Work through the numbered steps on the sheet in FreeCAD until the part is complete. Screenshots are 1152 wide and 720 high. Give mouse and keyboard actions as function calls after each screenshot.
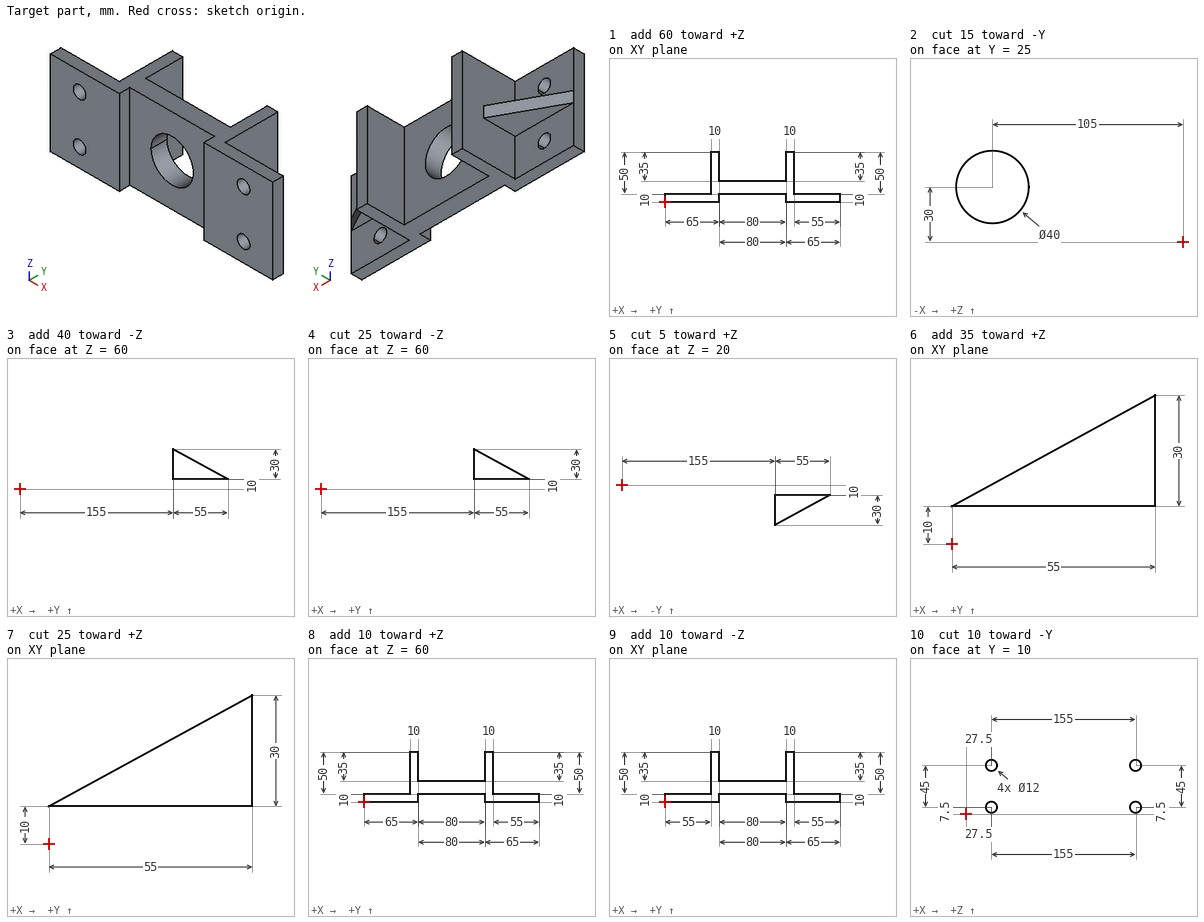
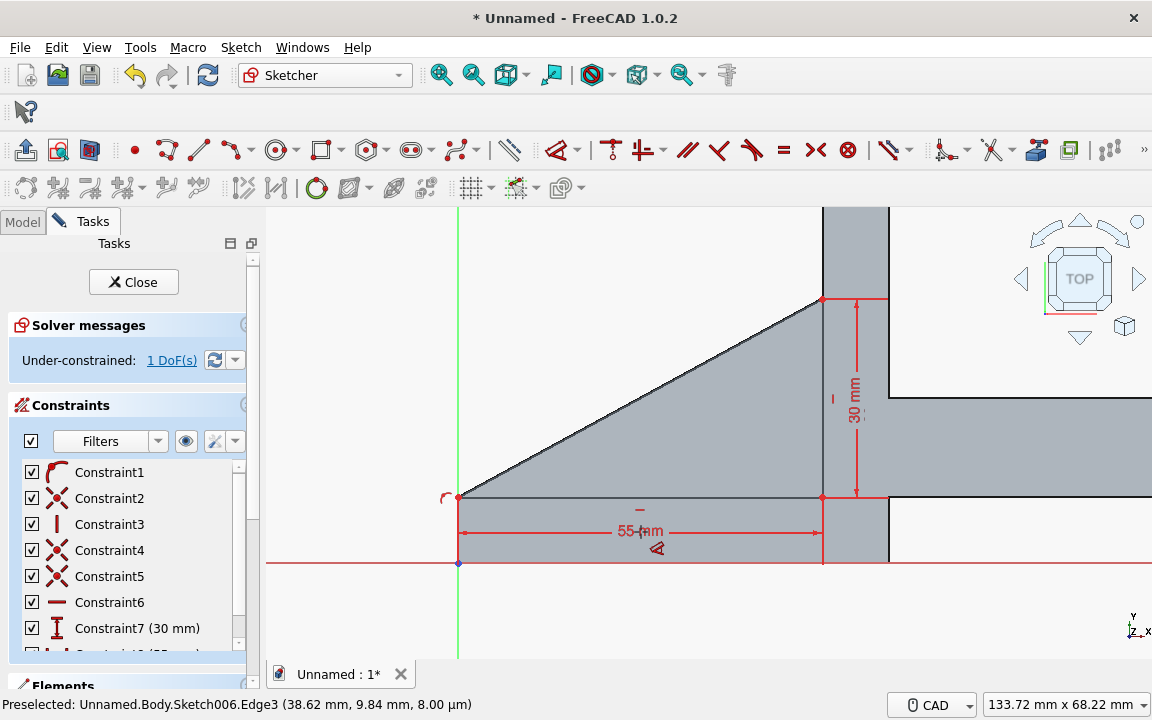
click(458, 498)
click(424, 531)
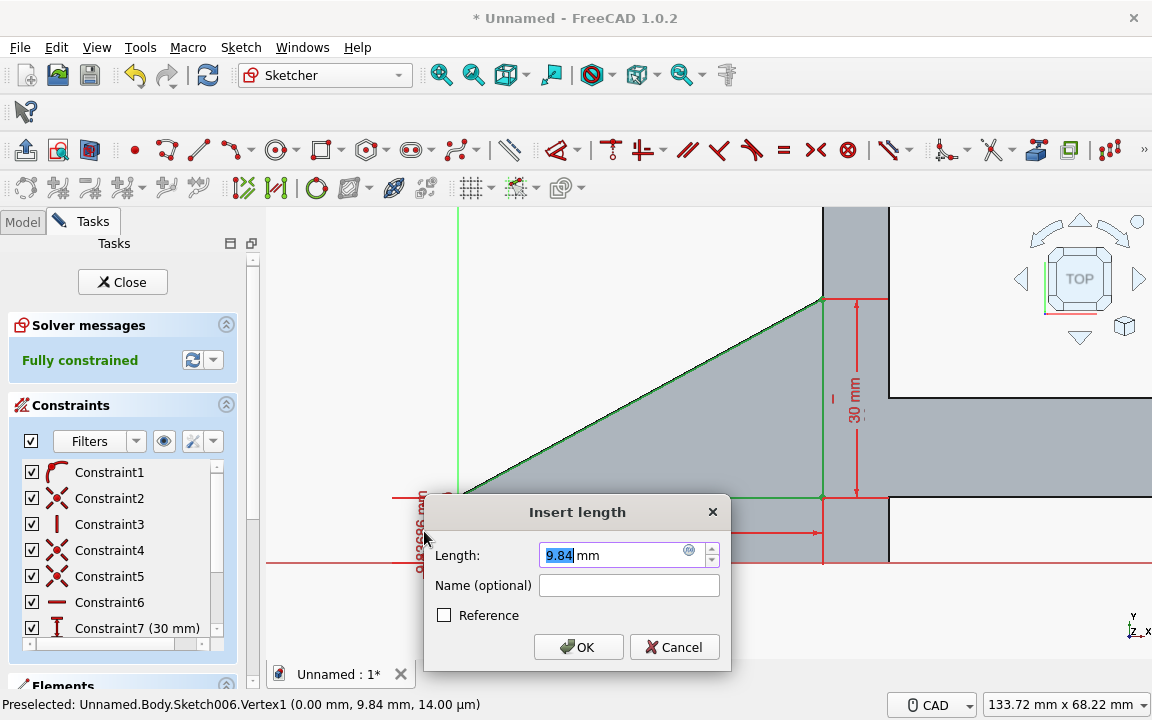
text(10)
key(Return)
key(Escape)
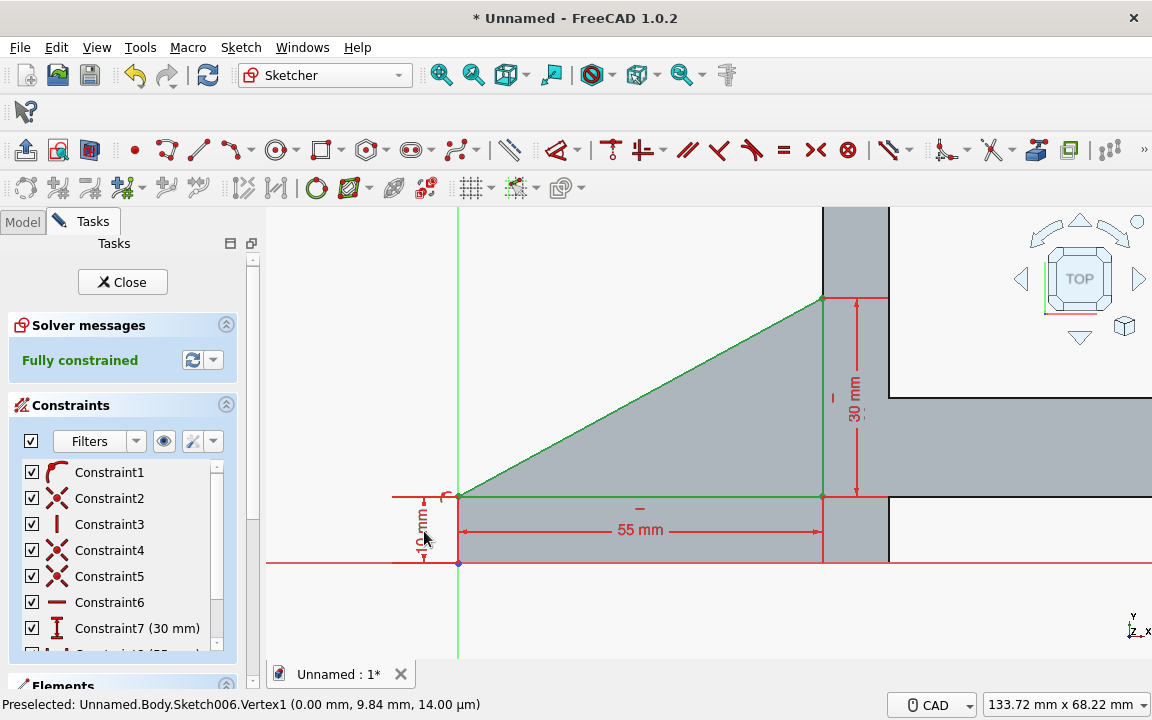
click(123, 282)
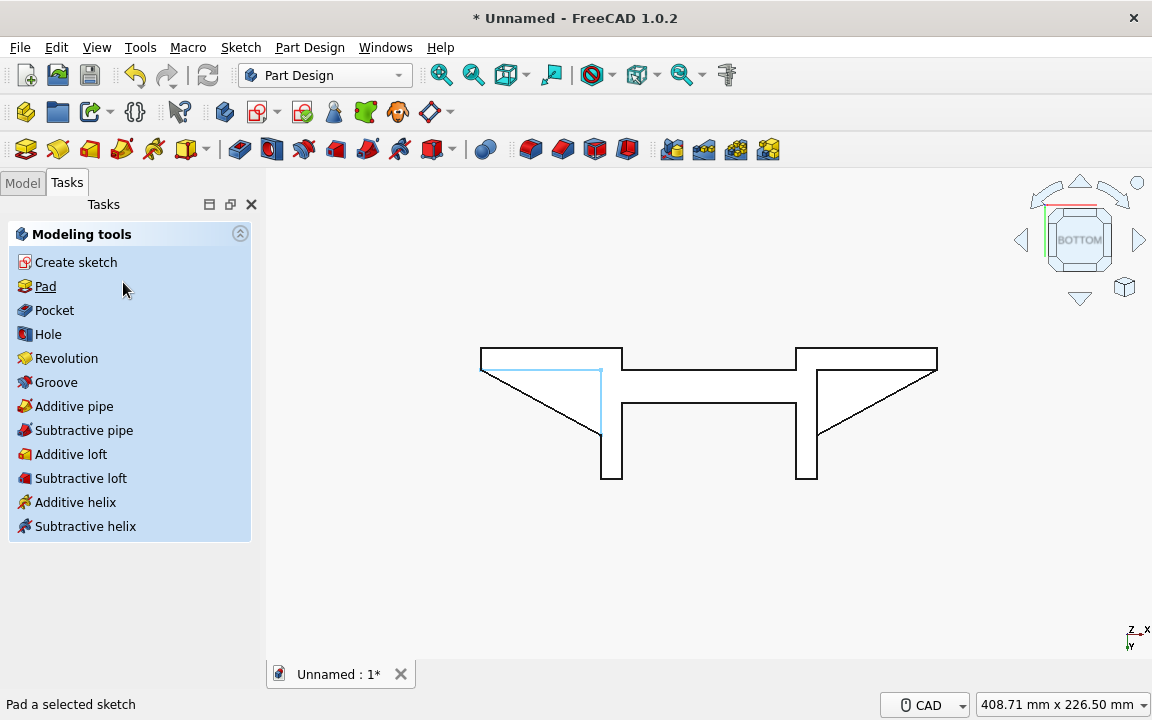
click(240, 150)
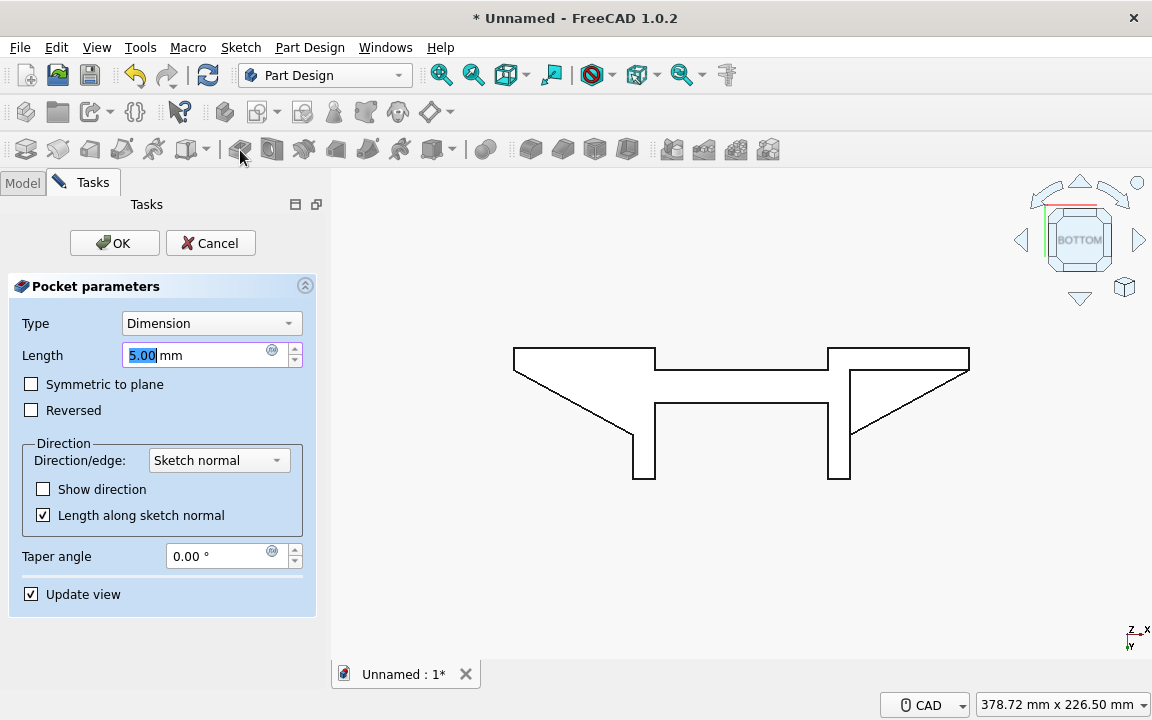
text(25)
key(Tab)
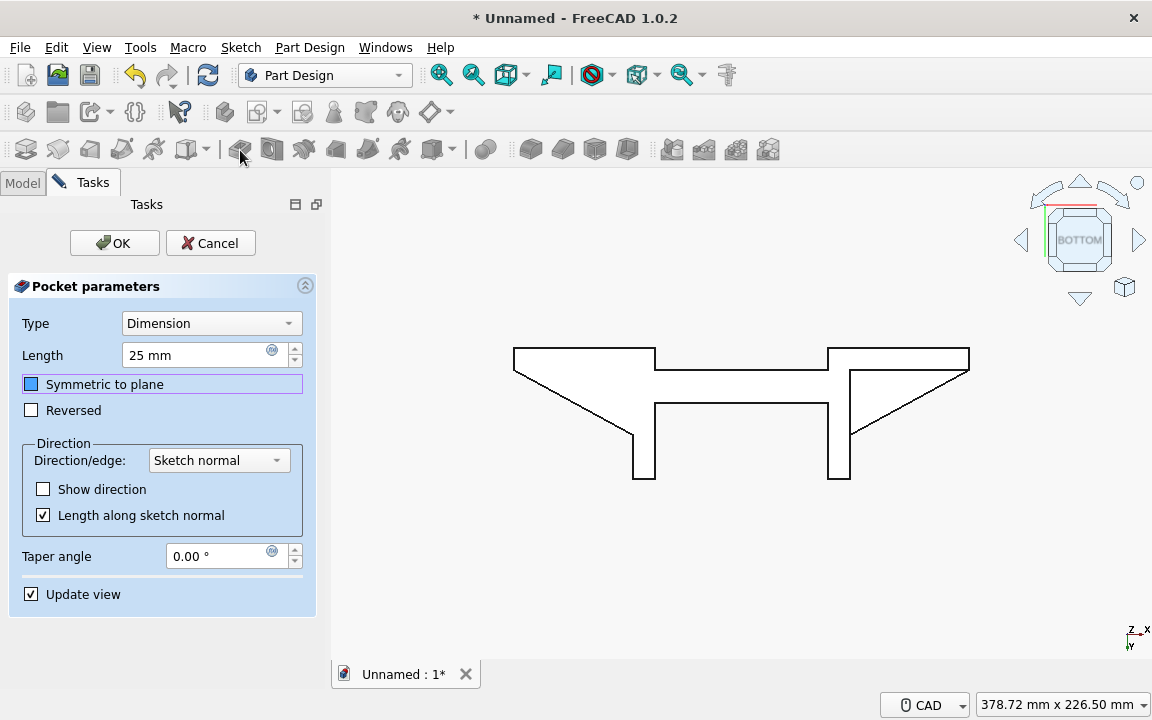
click(30, 410)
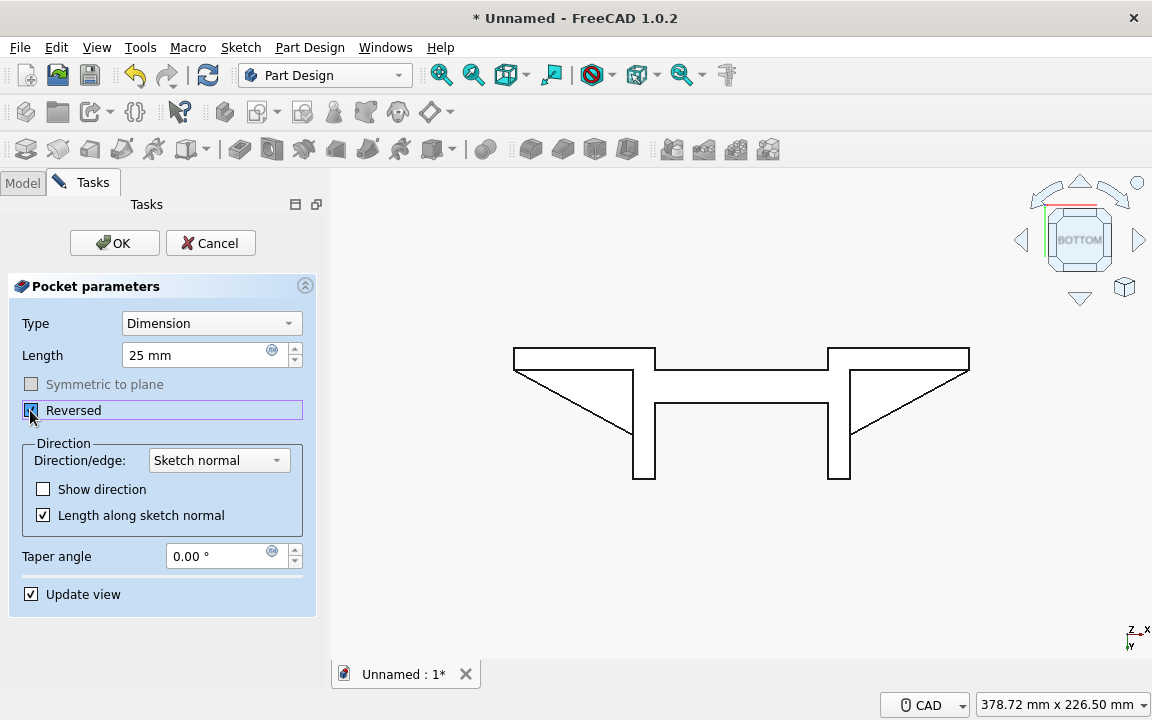
click(115, 243)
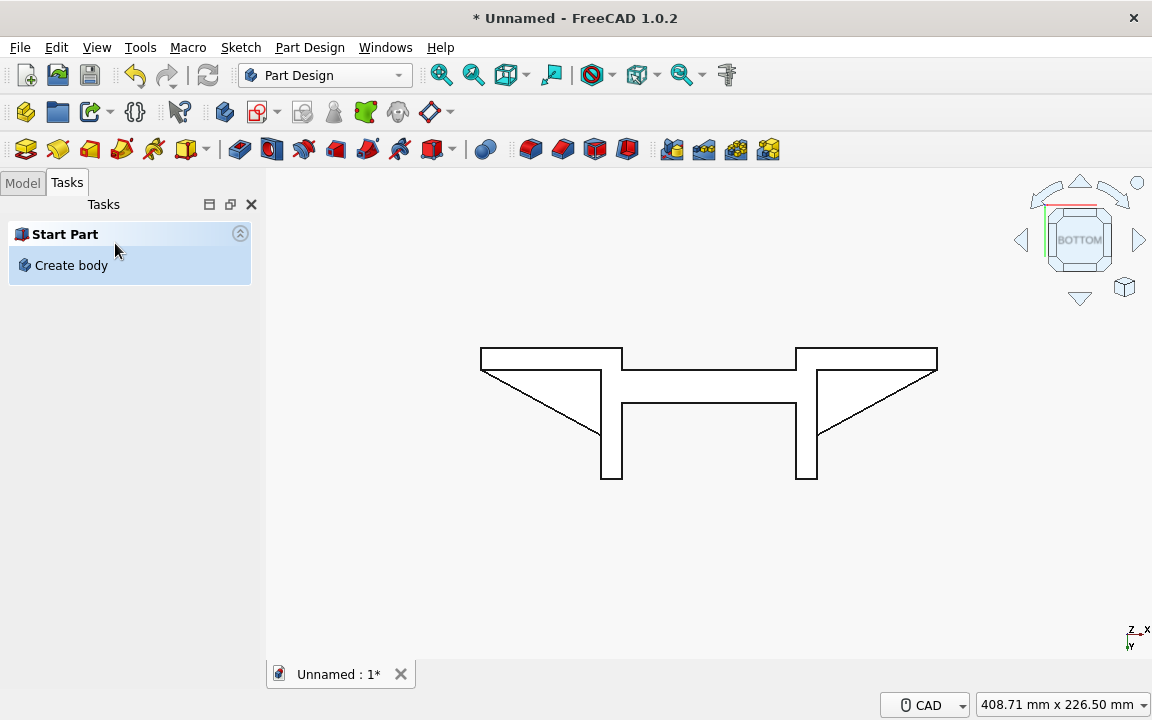
key(0)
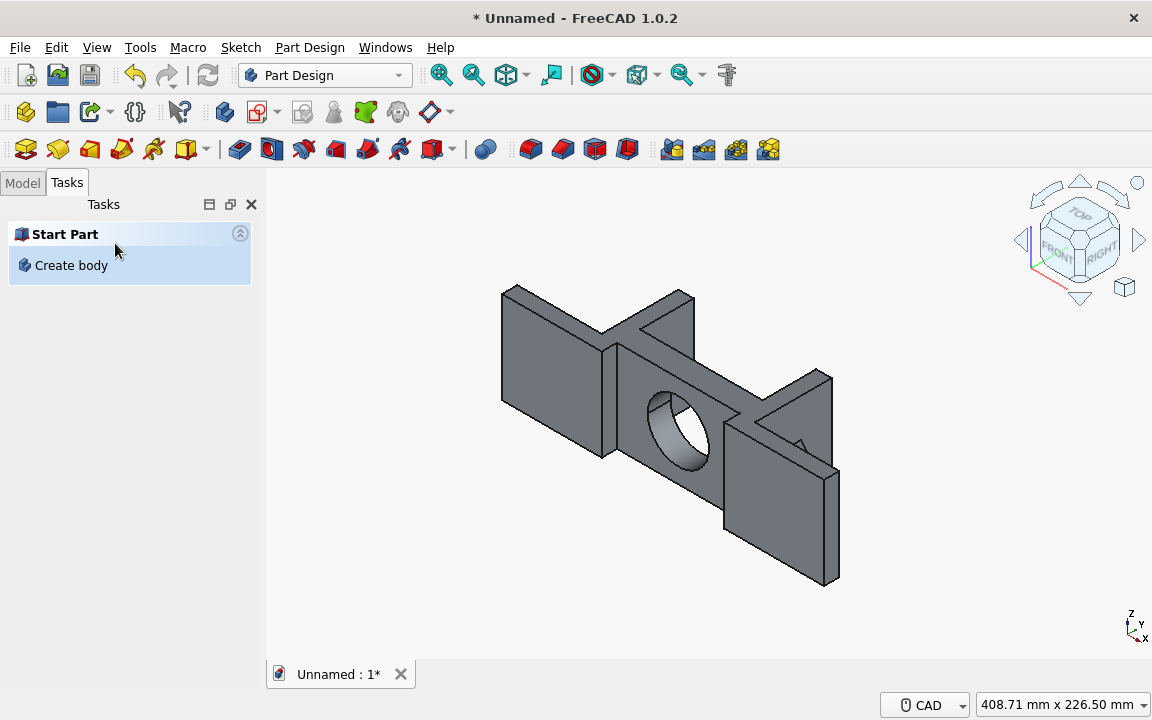
click(742, 394)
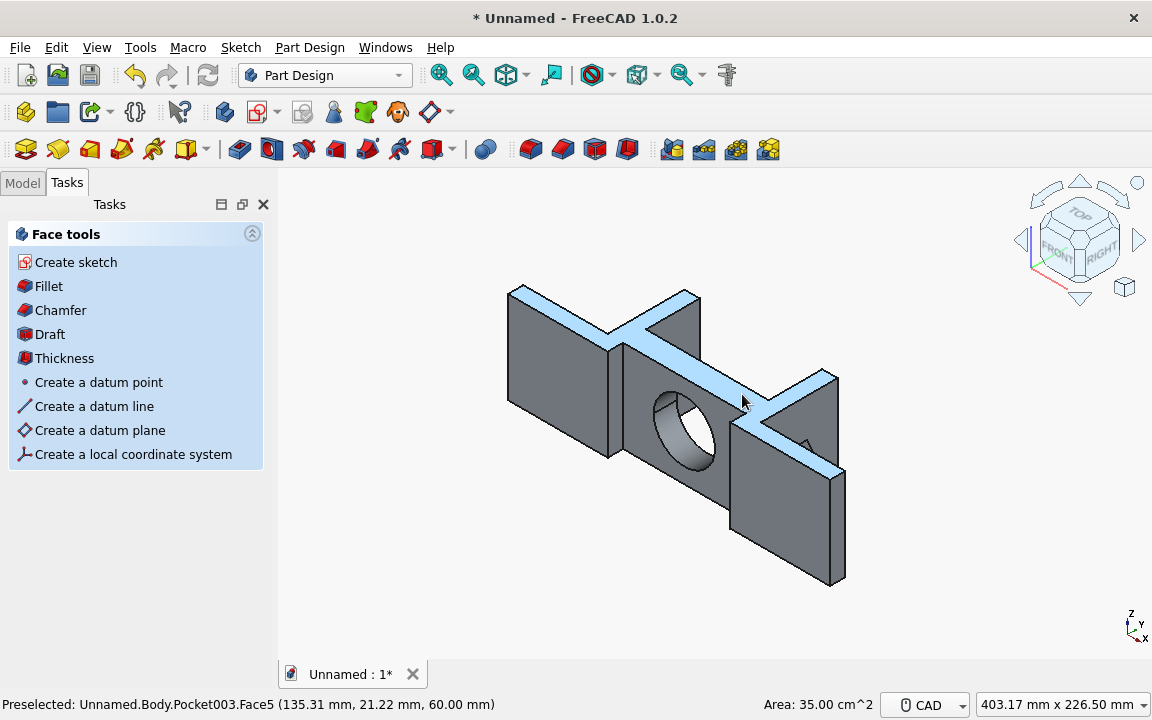
click(258, 112)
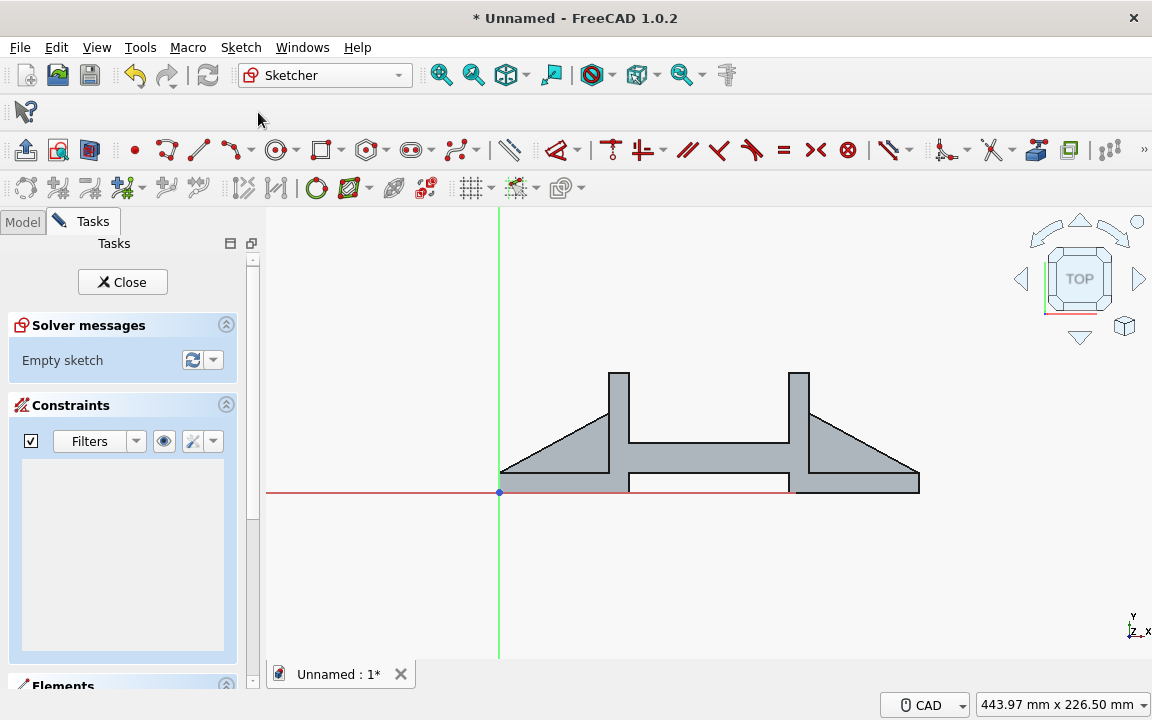
click(168, 150)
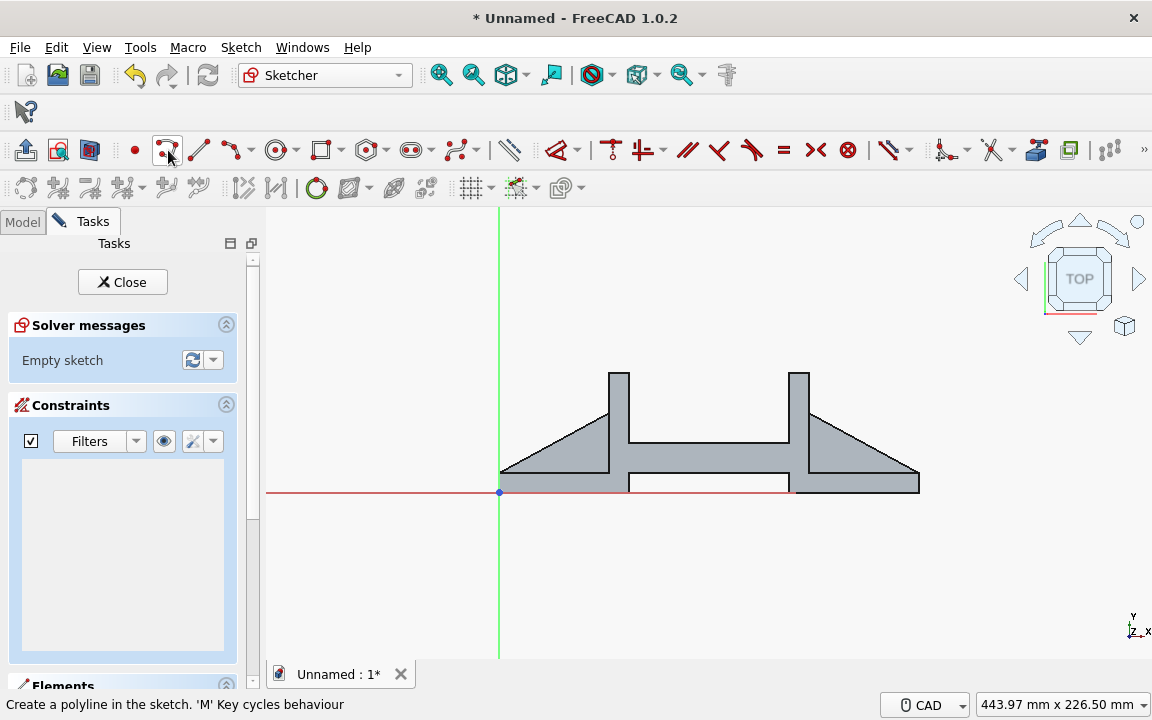
click(499, 493)
click(629, 484)
click(629, 473)
click(789, 473)
click(789, 493)
click(919, 484)
click(919, 473)
click(809, 473)
click(809, 373)
click(789, 373)
click(789, 443)
click(629, 443)
click(629, 373)
click(609, 373)
click(609, 473)
click(508, 473)
click(499, 493)
key(Escape)
key(Escape)